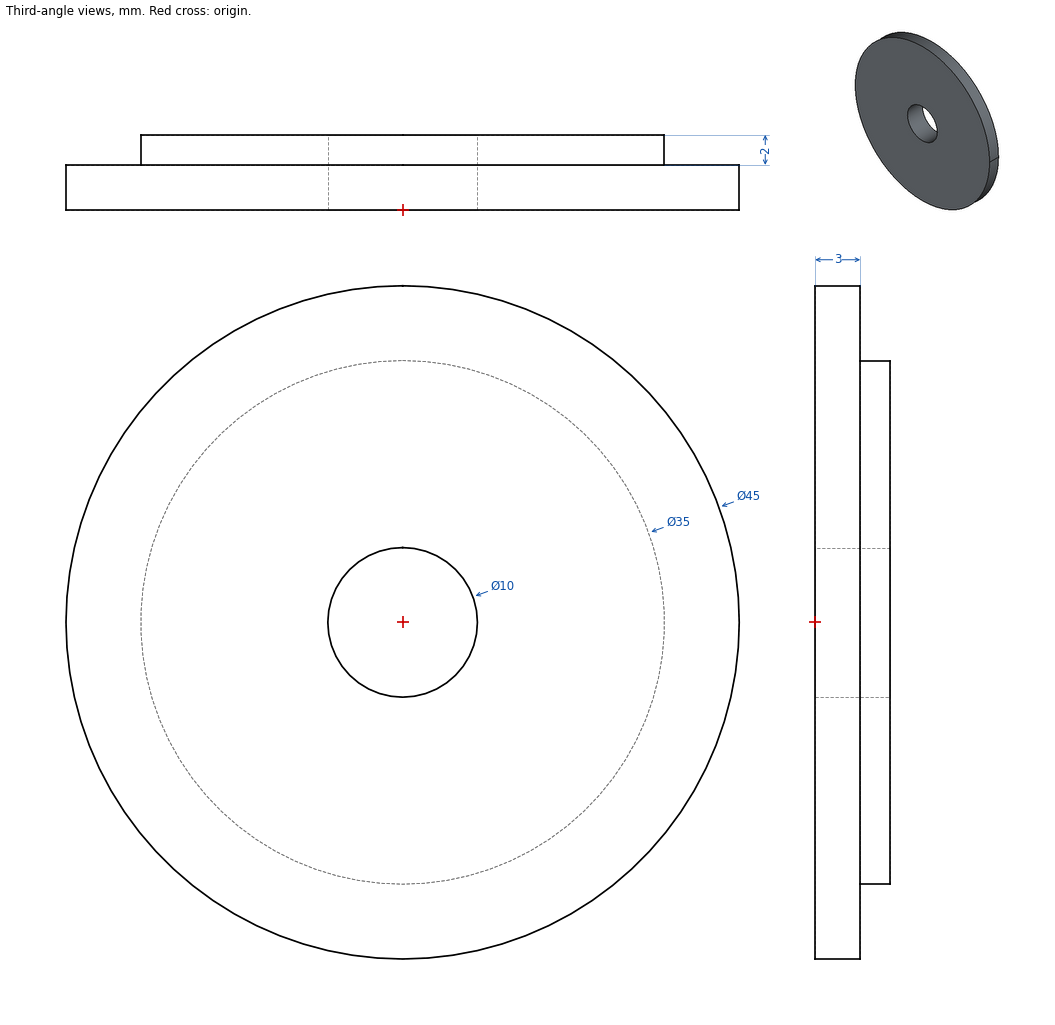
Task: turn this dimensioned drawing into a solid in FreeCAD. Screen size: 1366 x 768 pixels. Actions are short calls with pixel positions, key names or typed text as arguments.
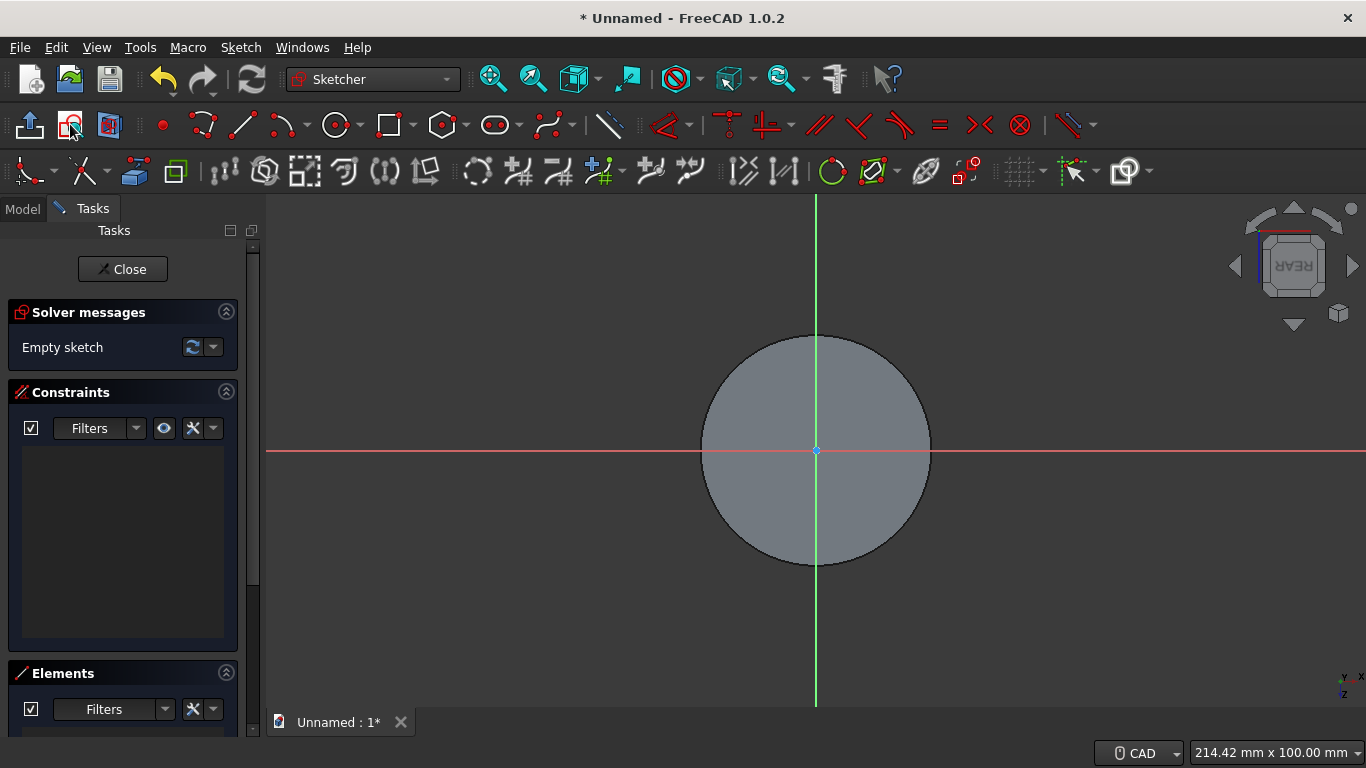
scroll(899, 451, up, 3)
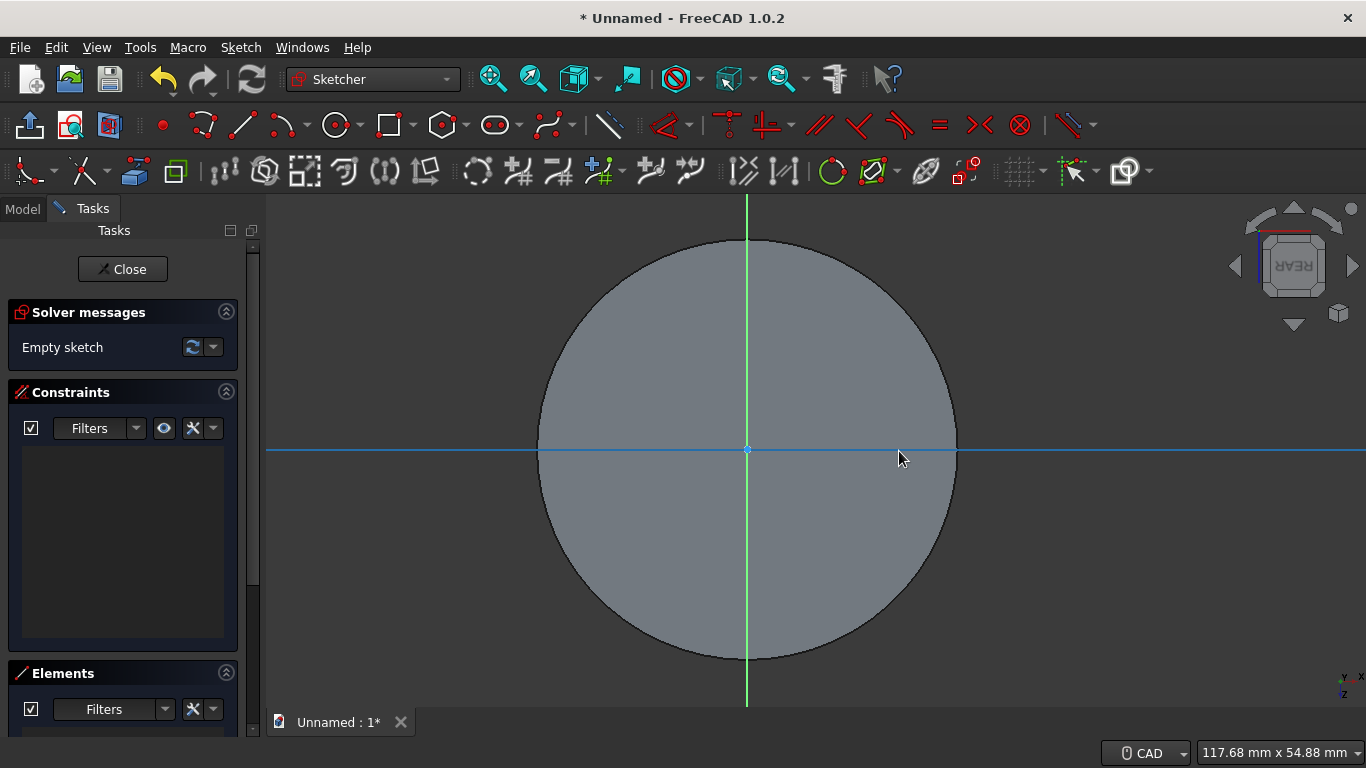
key(g)
key(c)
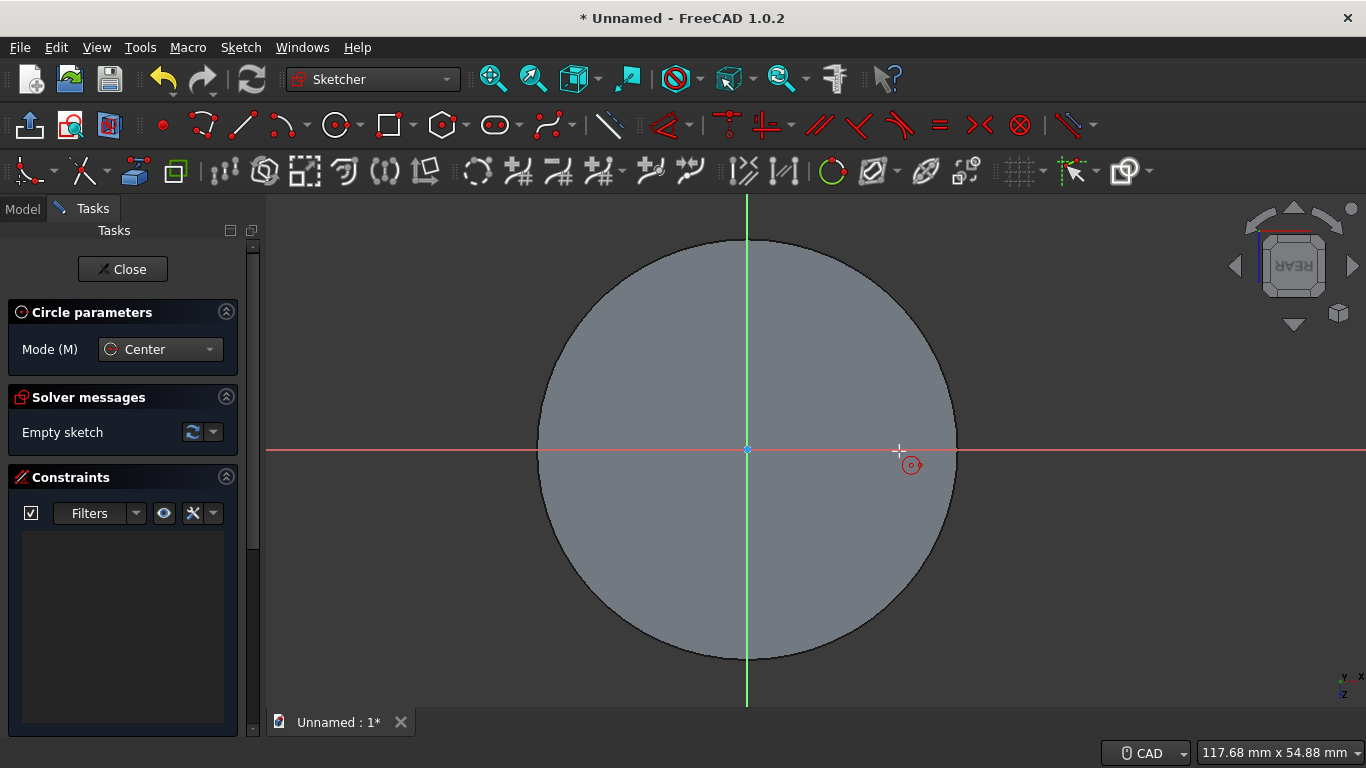
click(747, 450)
click(863, 334)
key(Escape)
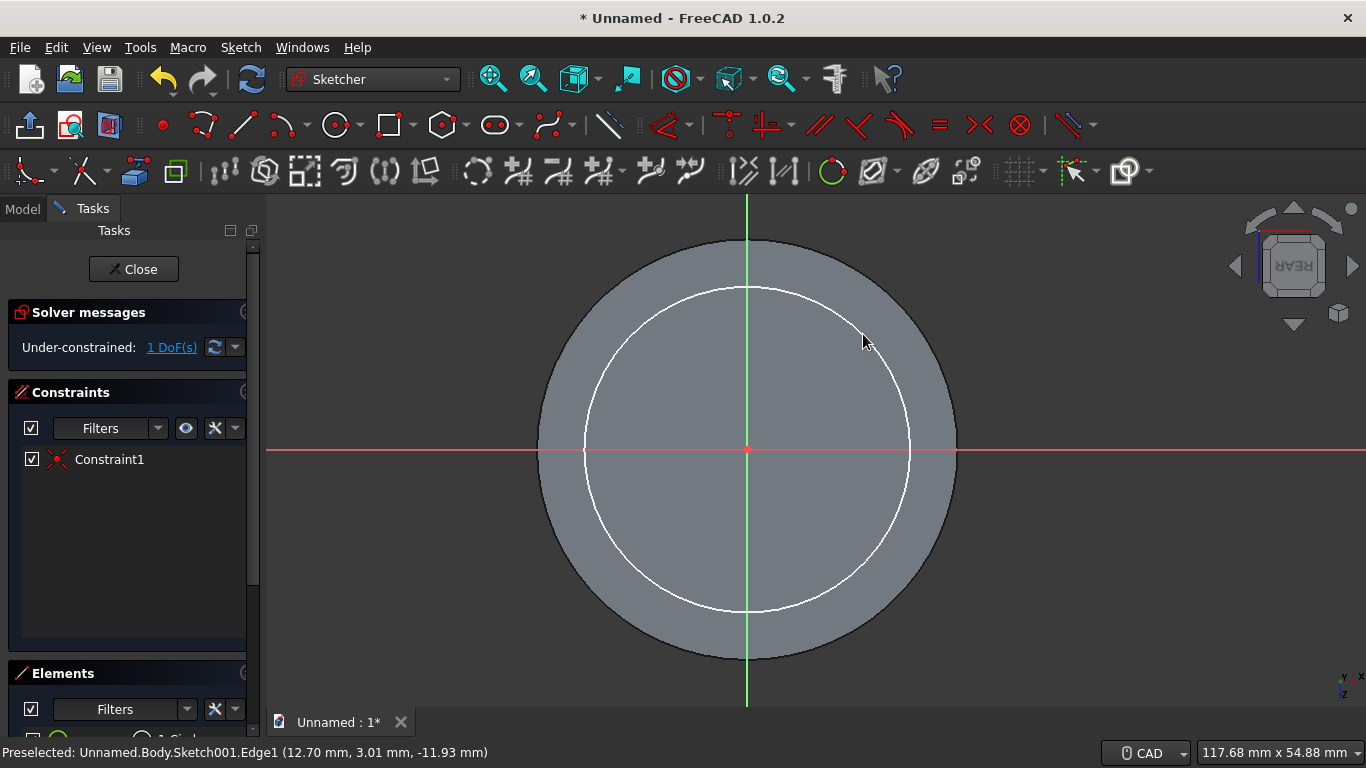
key(d)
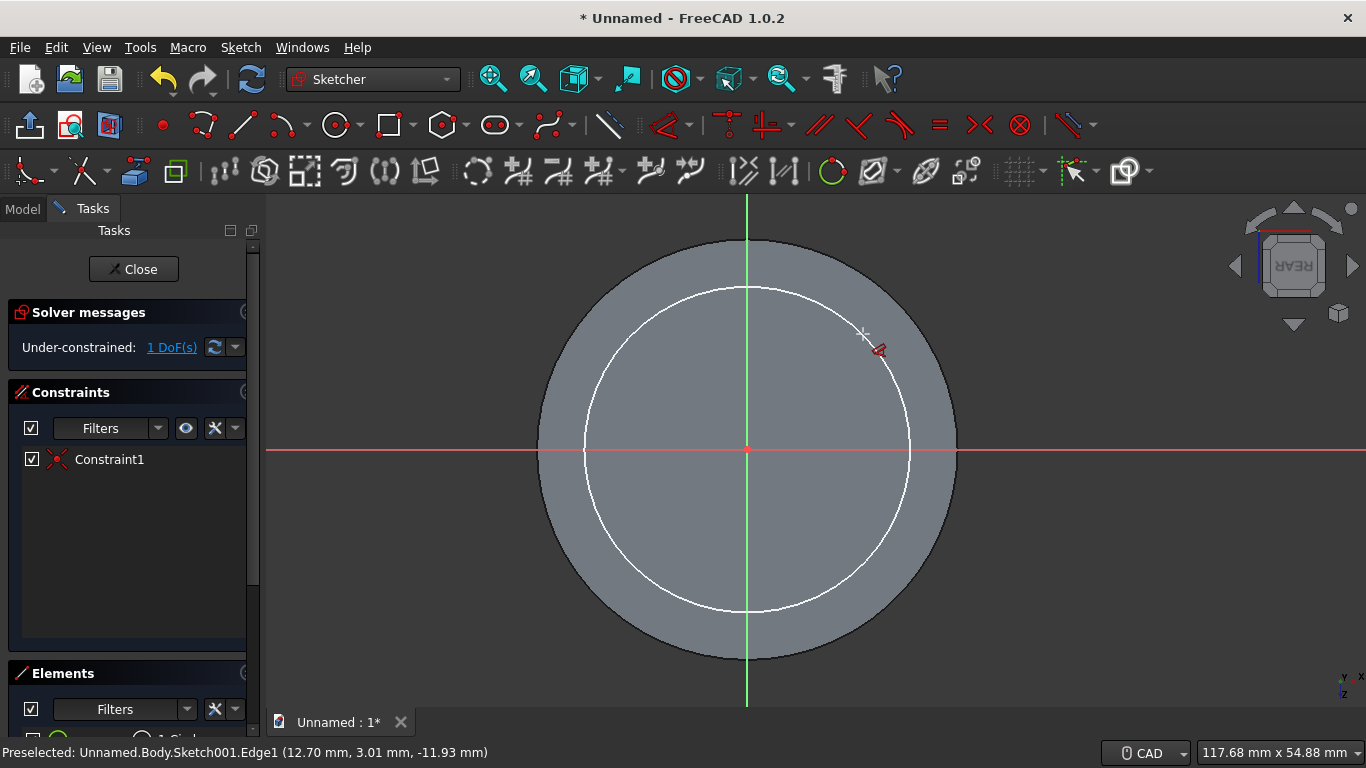
click(862, 334)
click(885, 311)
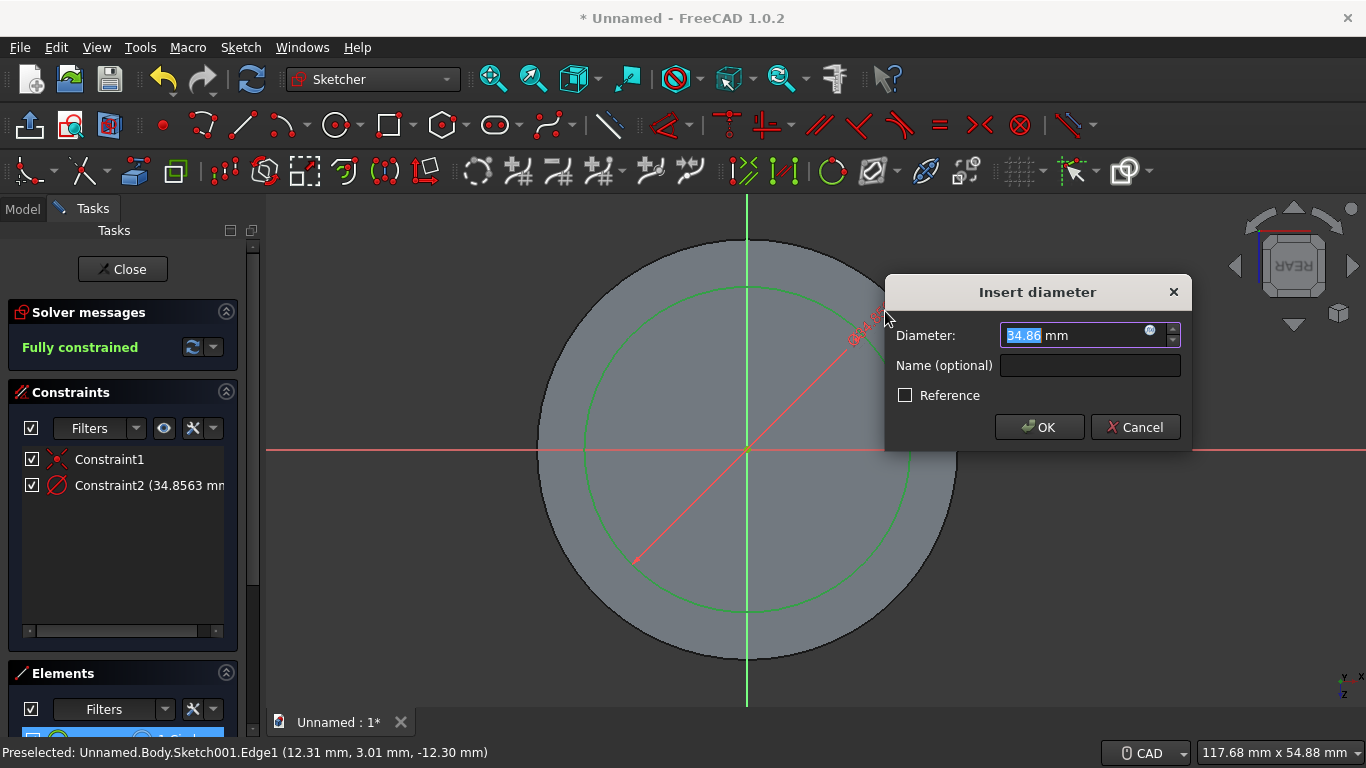
text(35)
key(Return)
key(Escape)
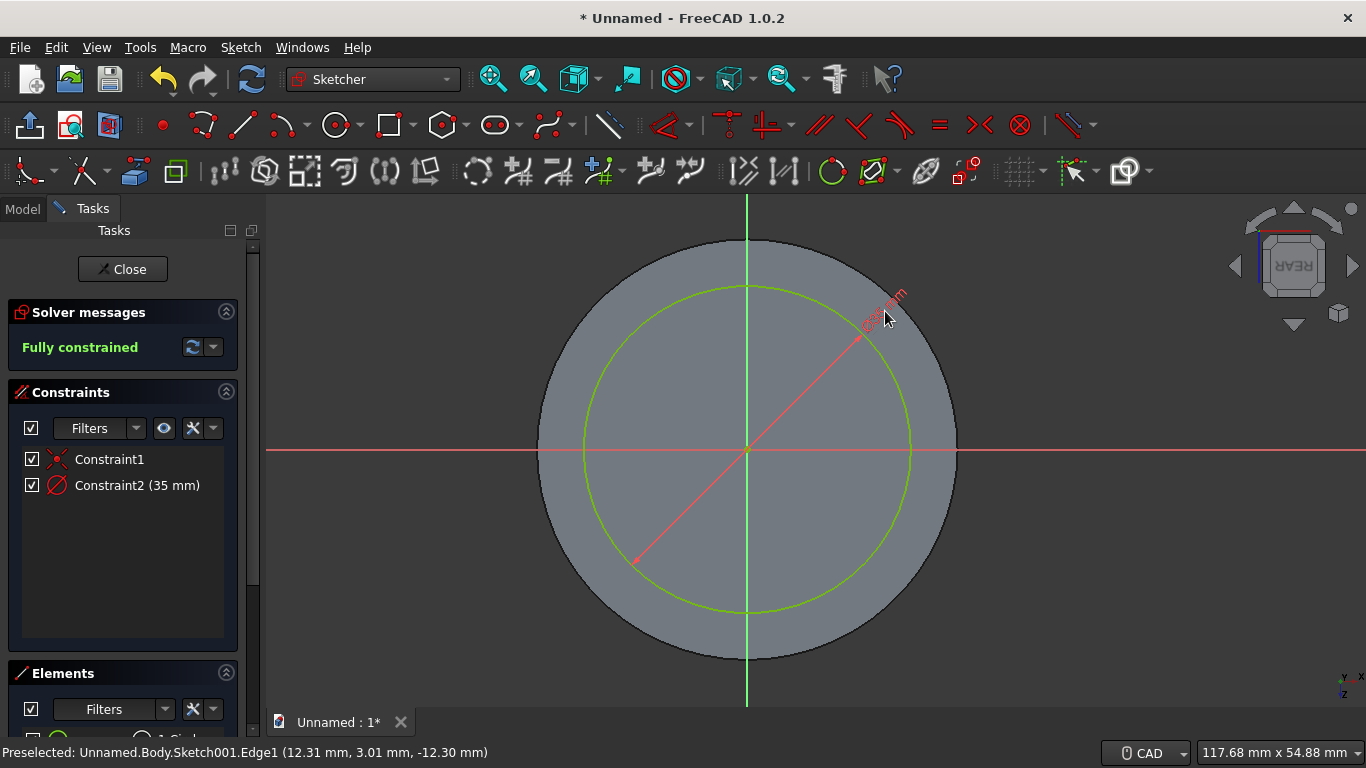
click(123, 269)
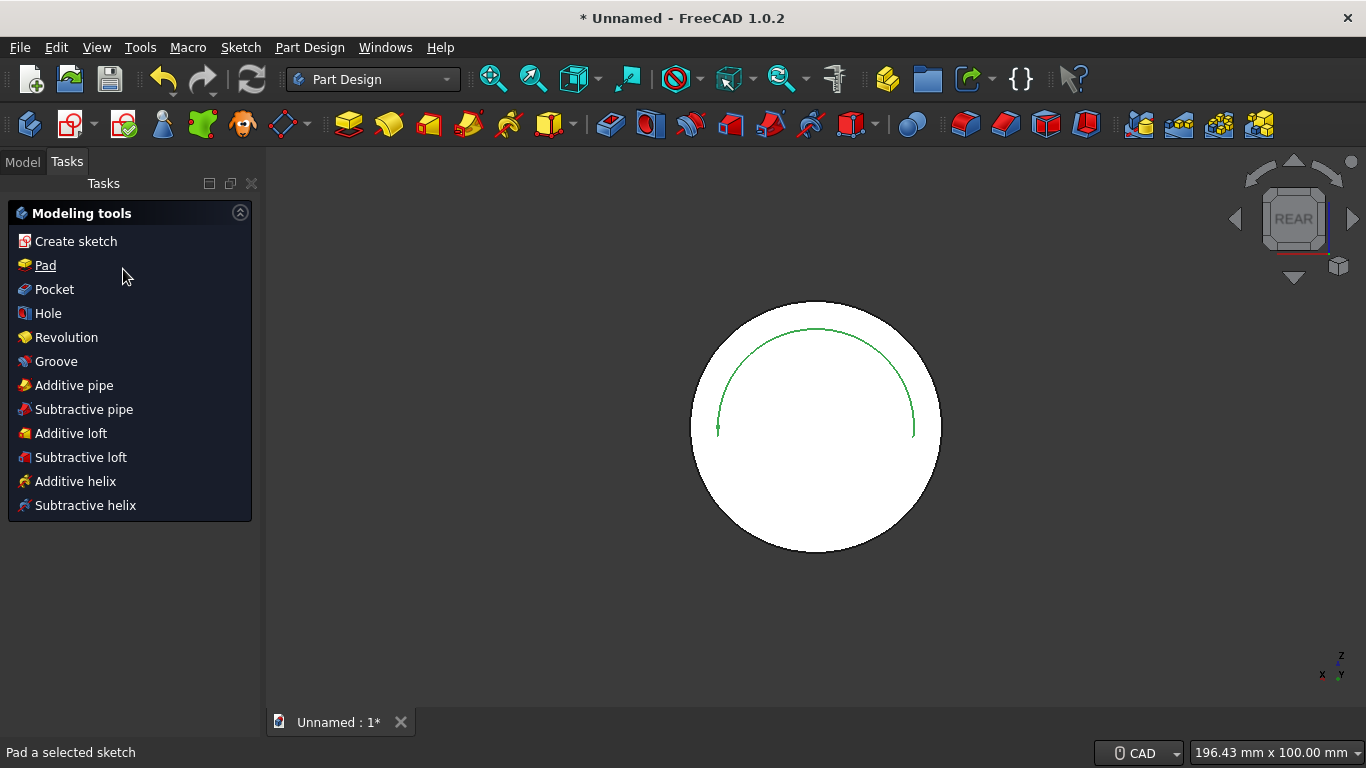
click(350, 124)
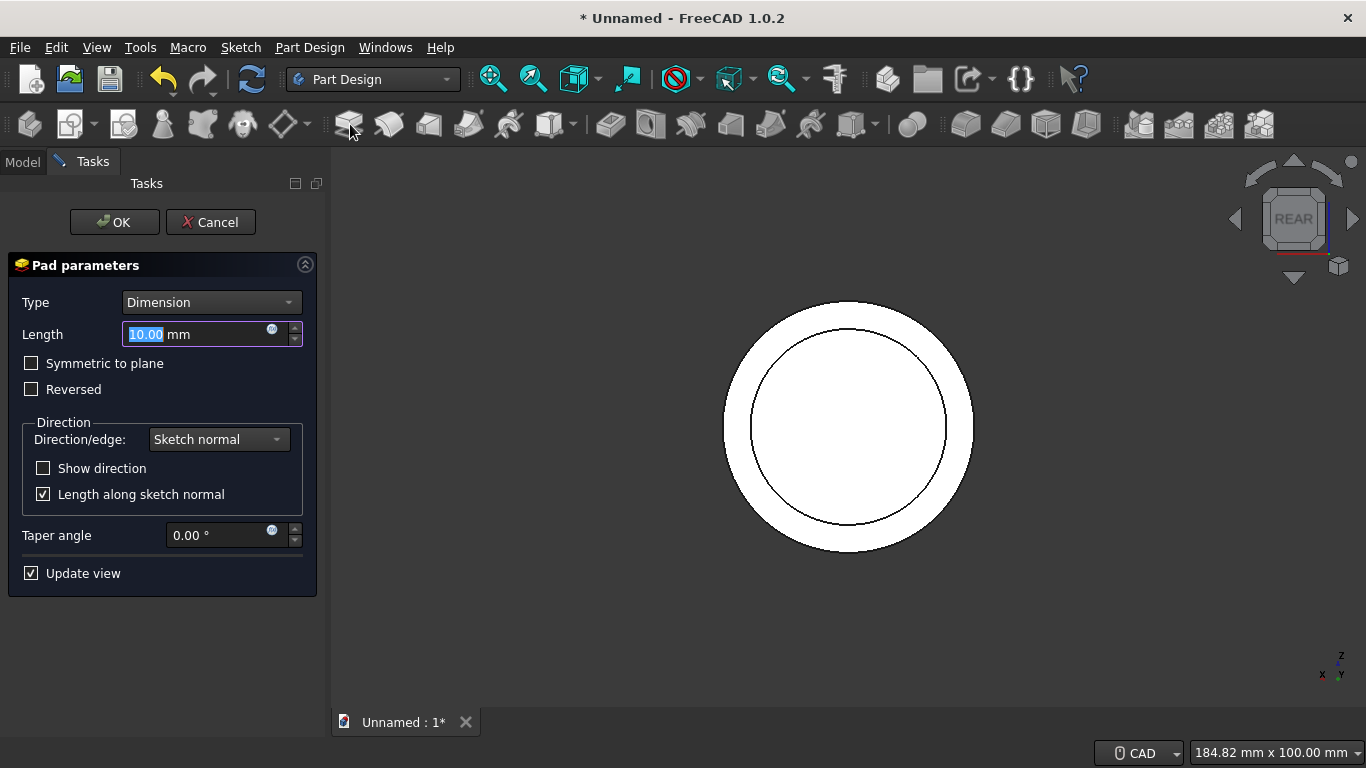
text(2)
key(Tab)